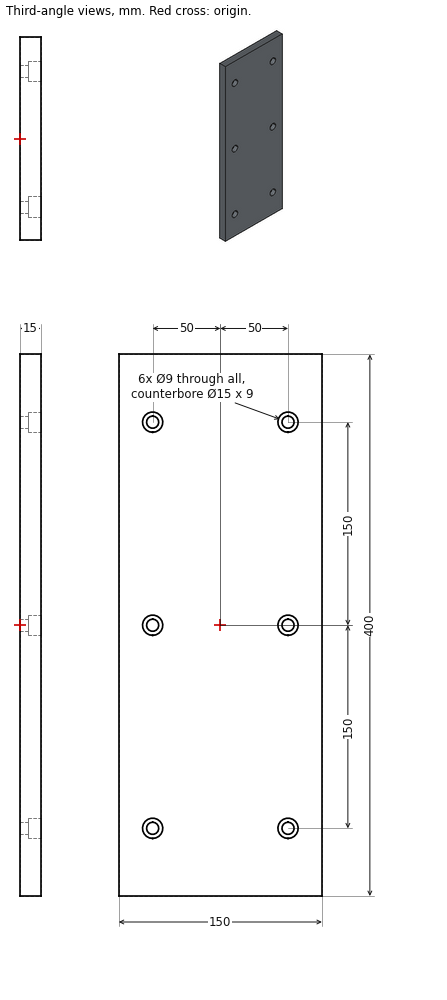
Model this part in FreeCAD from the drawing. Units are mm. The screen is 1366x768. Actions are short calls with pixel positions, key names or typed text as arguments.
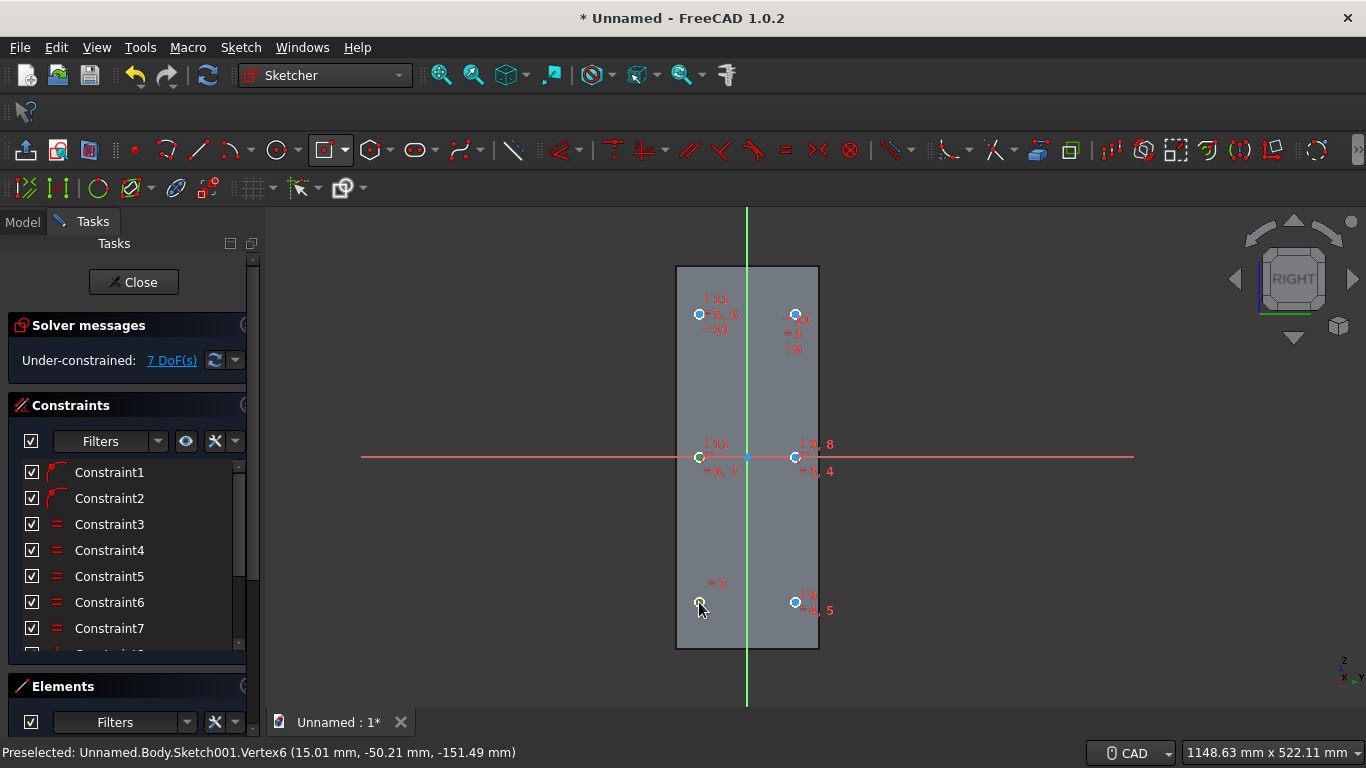
key(v)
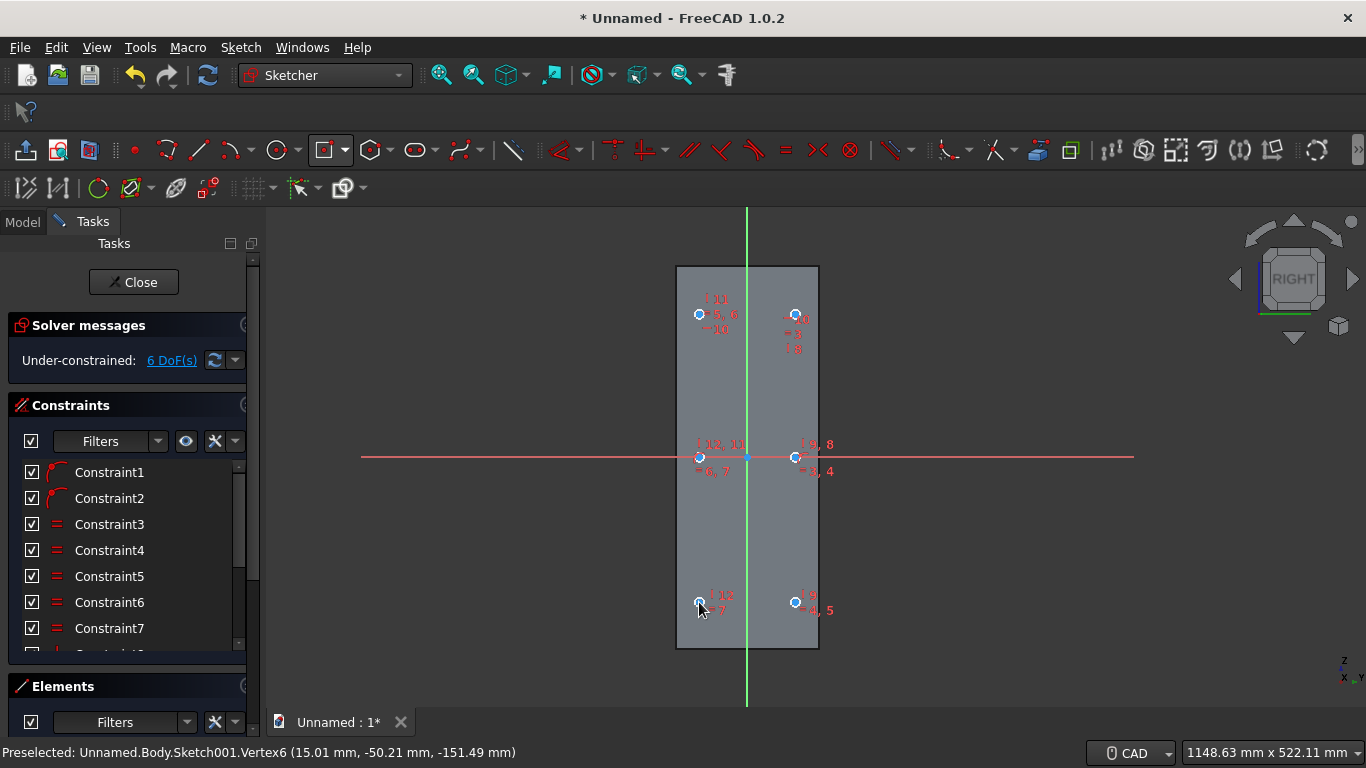
click(795, 602)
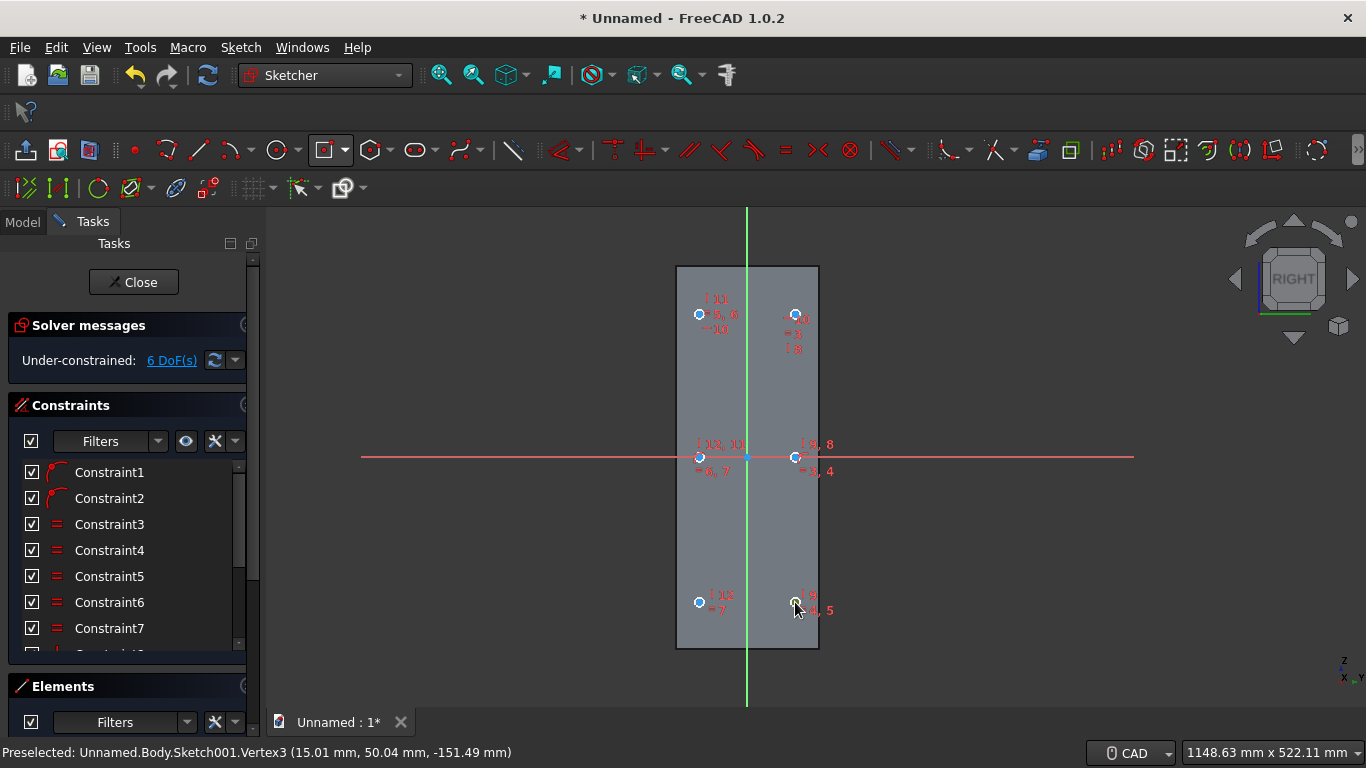
click(699, 602)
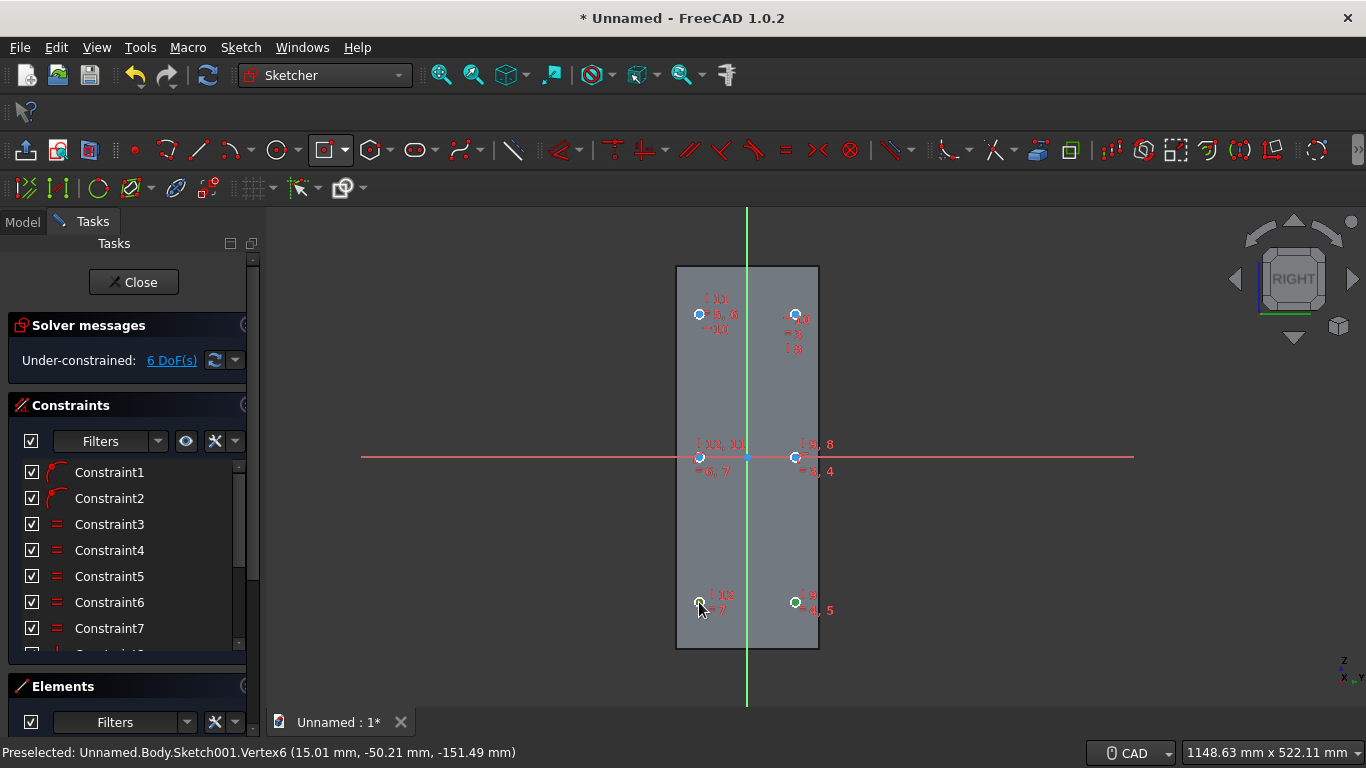
key(h)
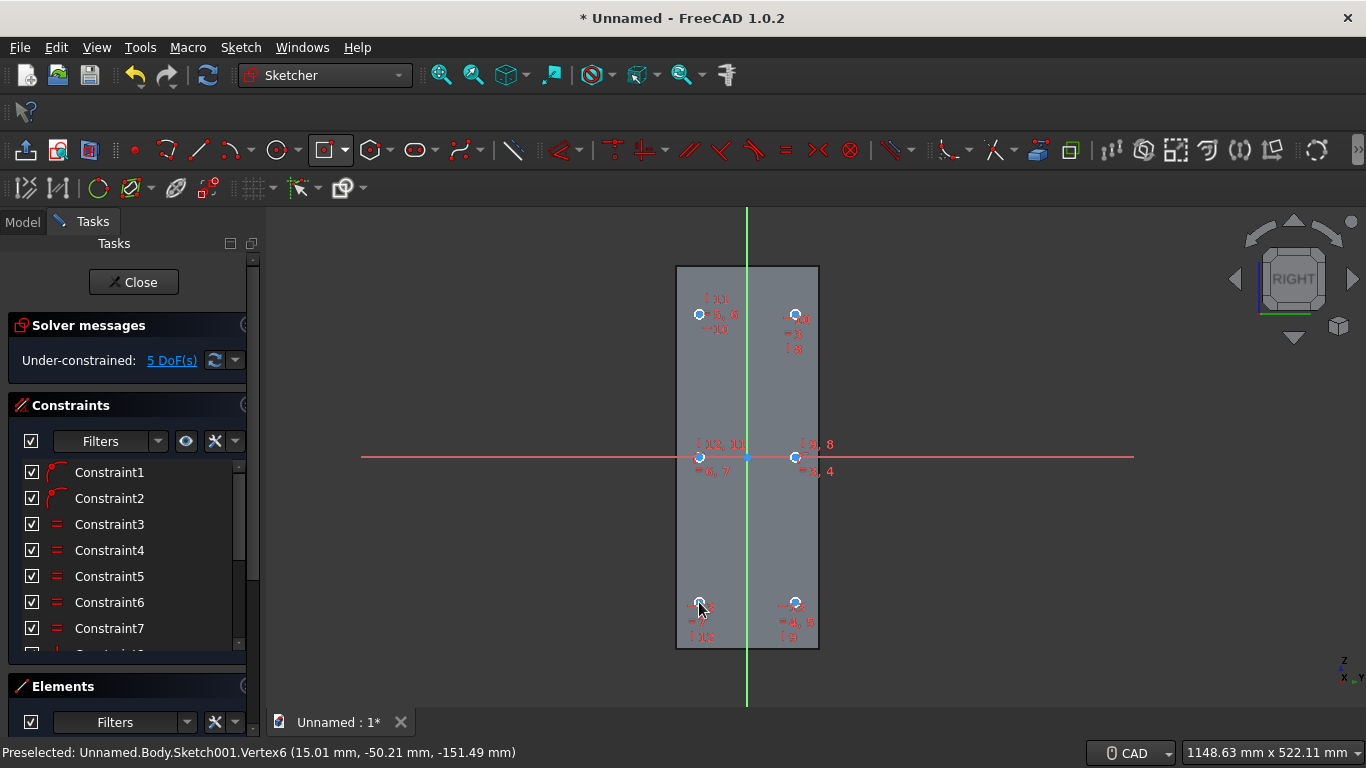
key(d)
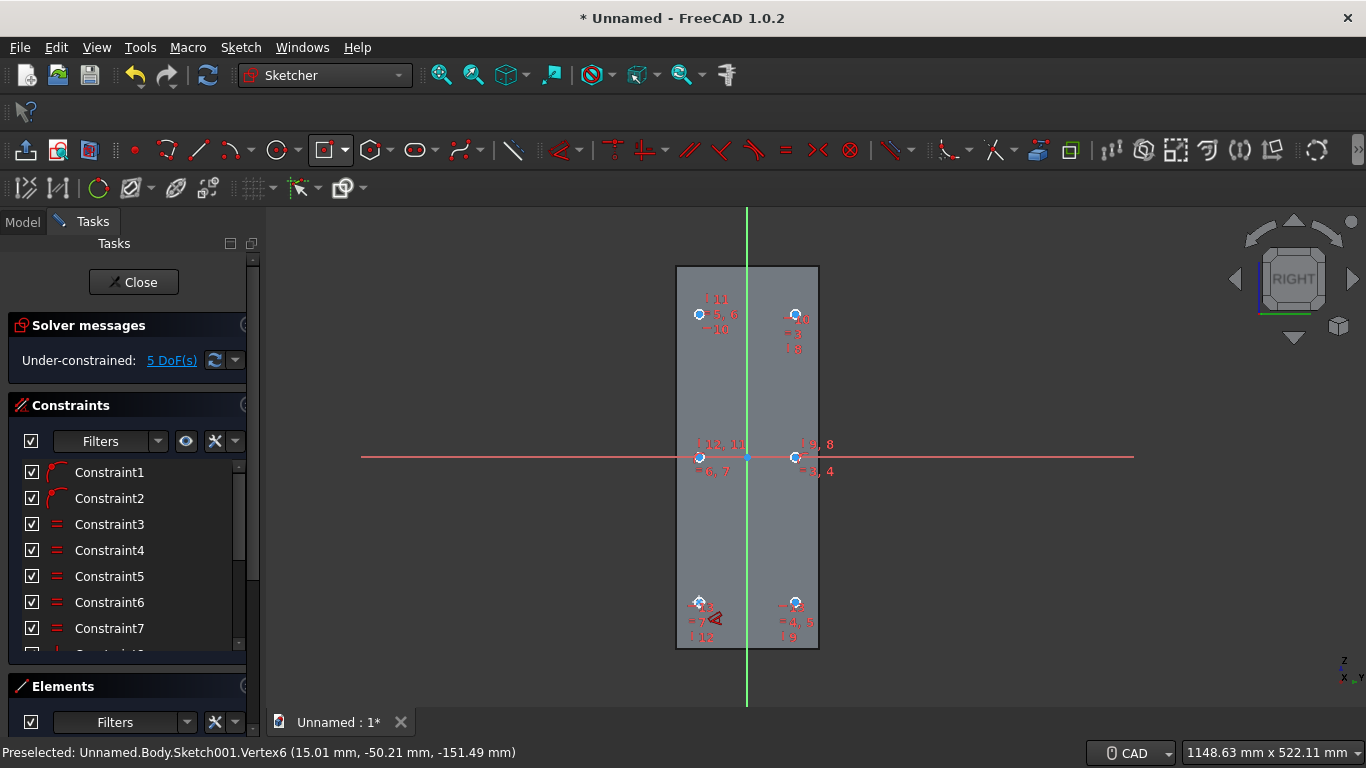
scroll(792, 311, up, 8)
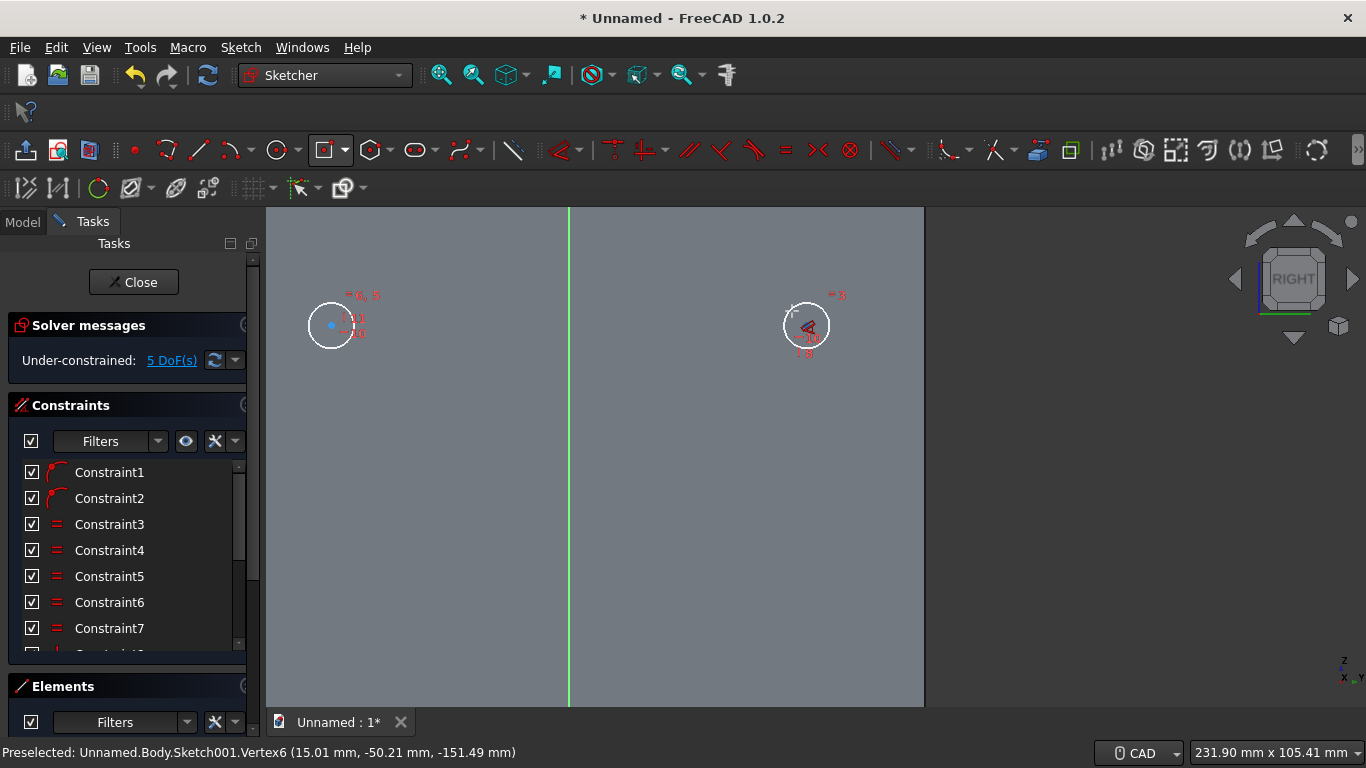
click(791, 310)
click(768, 287)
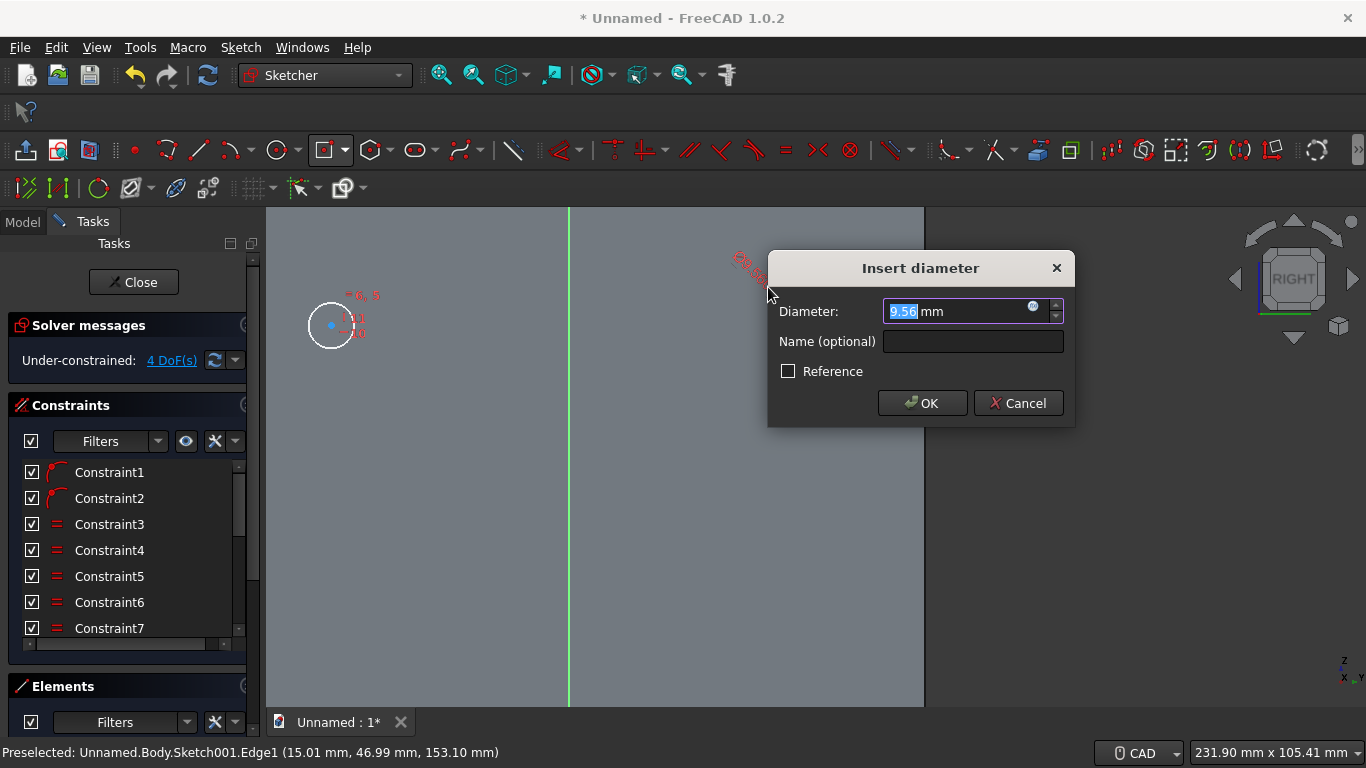
text(9)
key(Return)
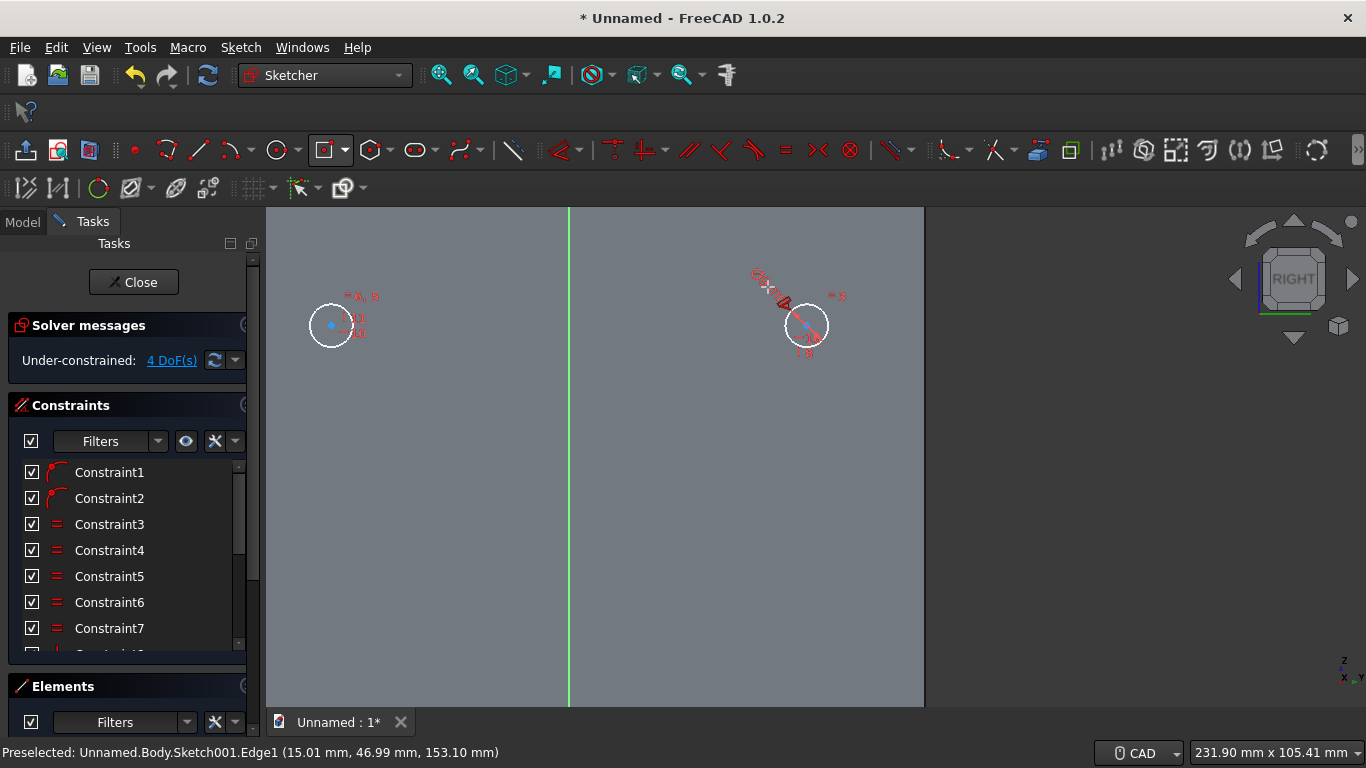
scroll(793, 311, down, 8)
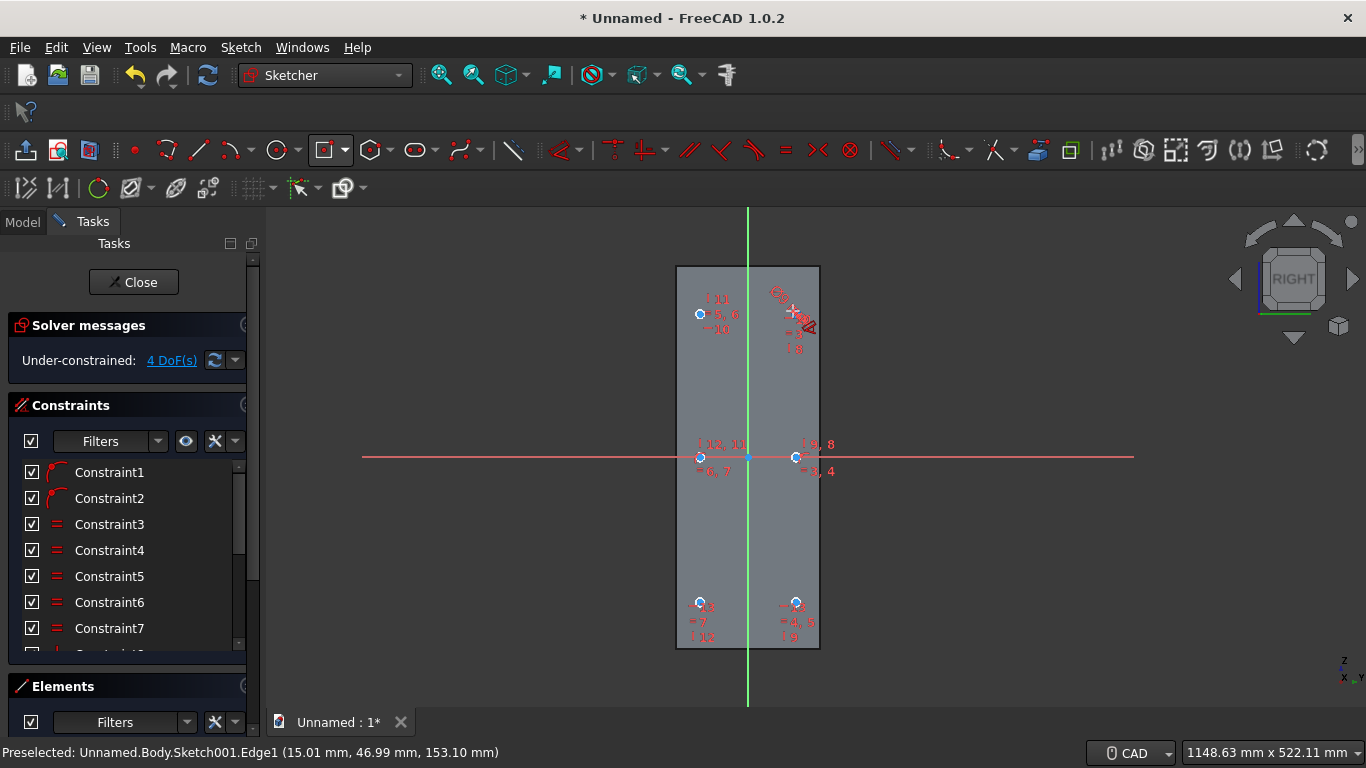
click(796, 314)
click(772, 280)